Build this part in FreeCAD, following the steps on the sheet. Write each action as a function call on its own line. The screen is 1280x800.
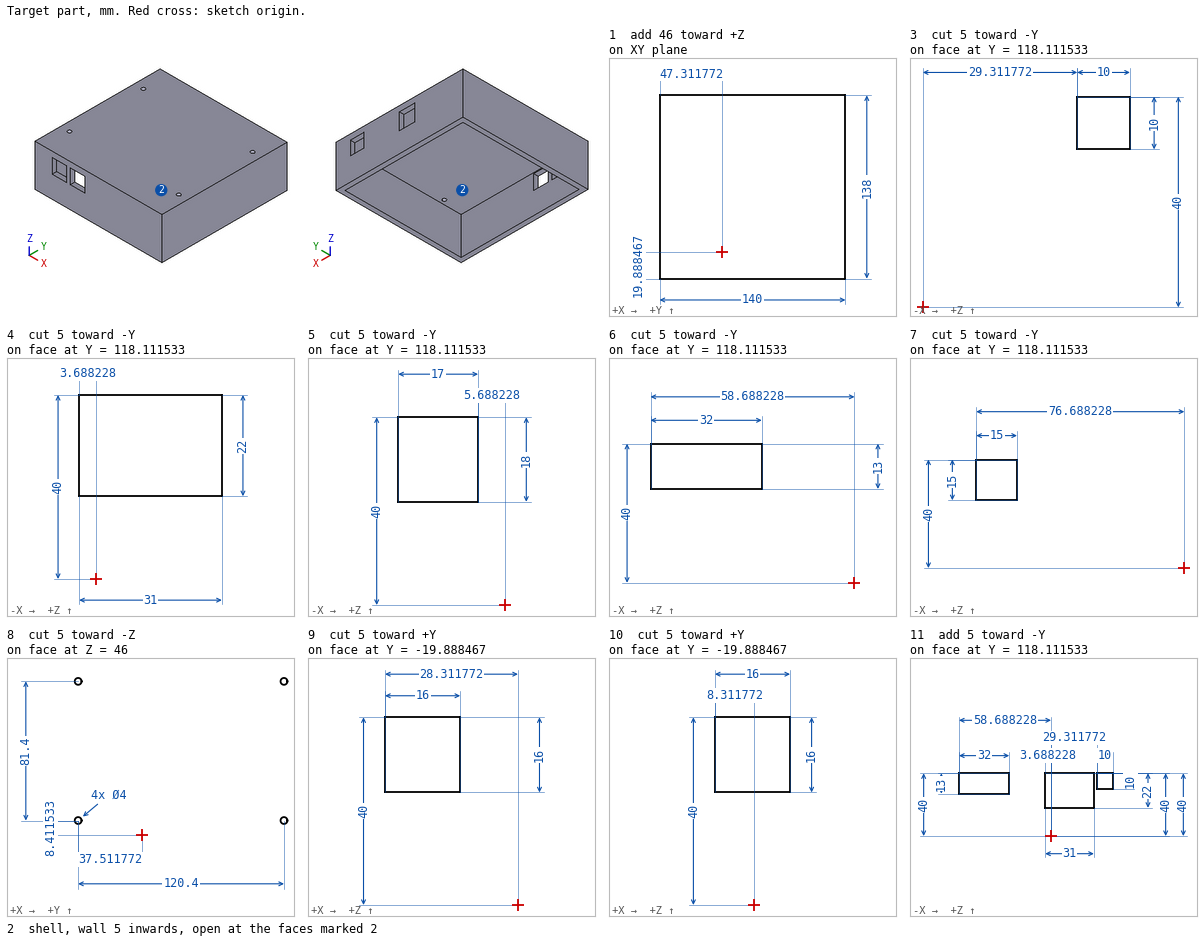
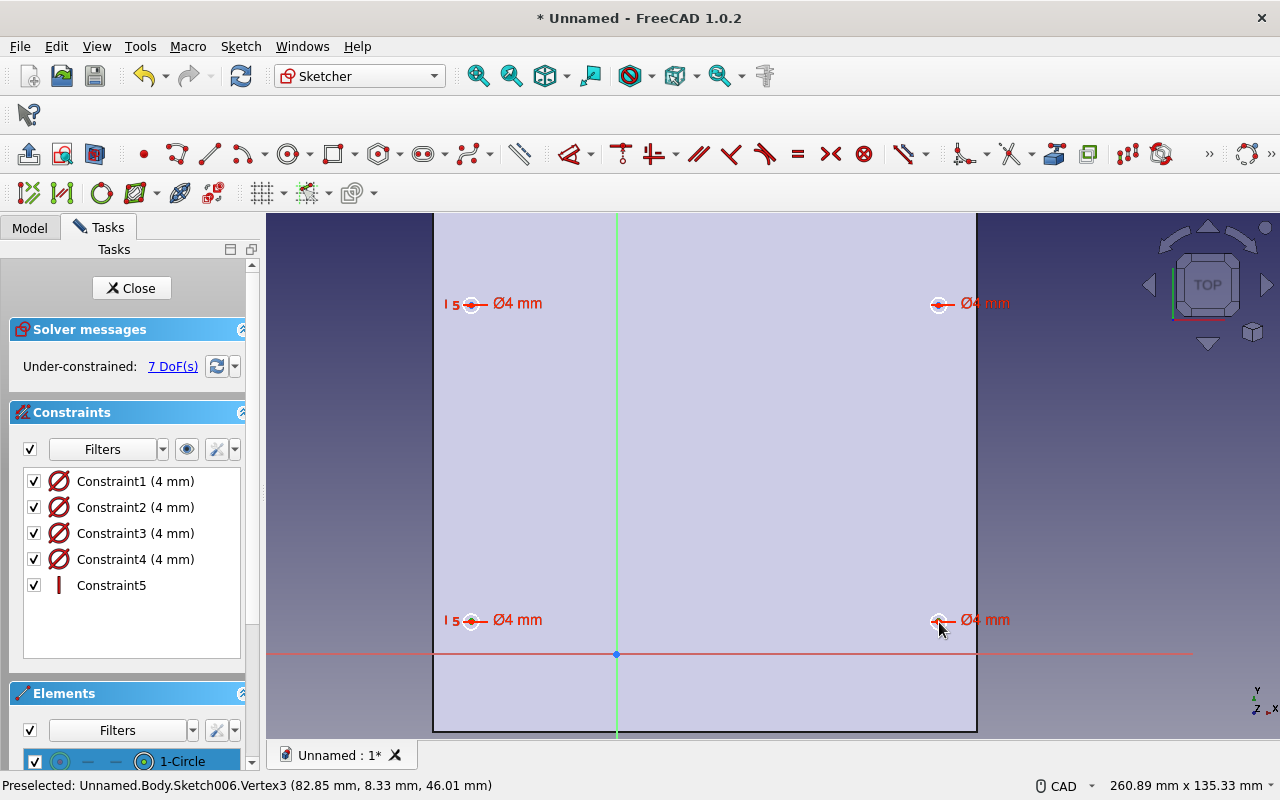
key(h)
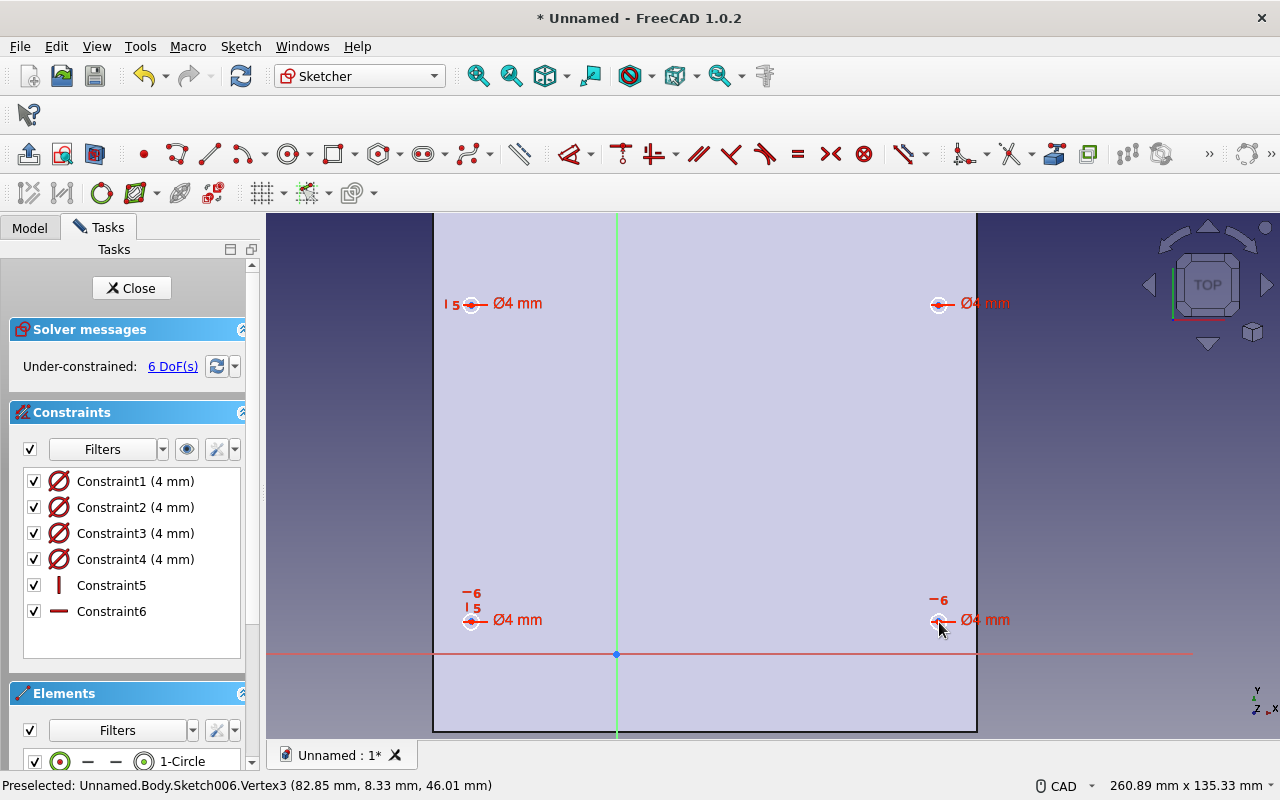
click(939, 622)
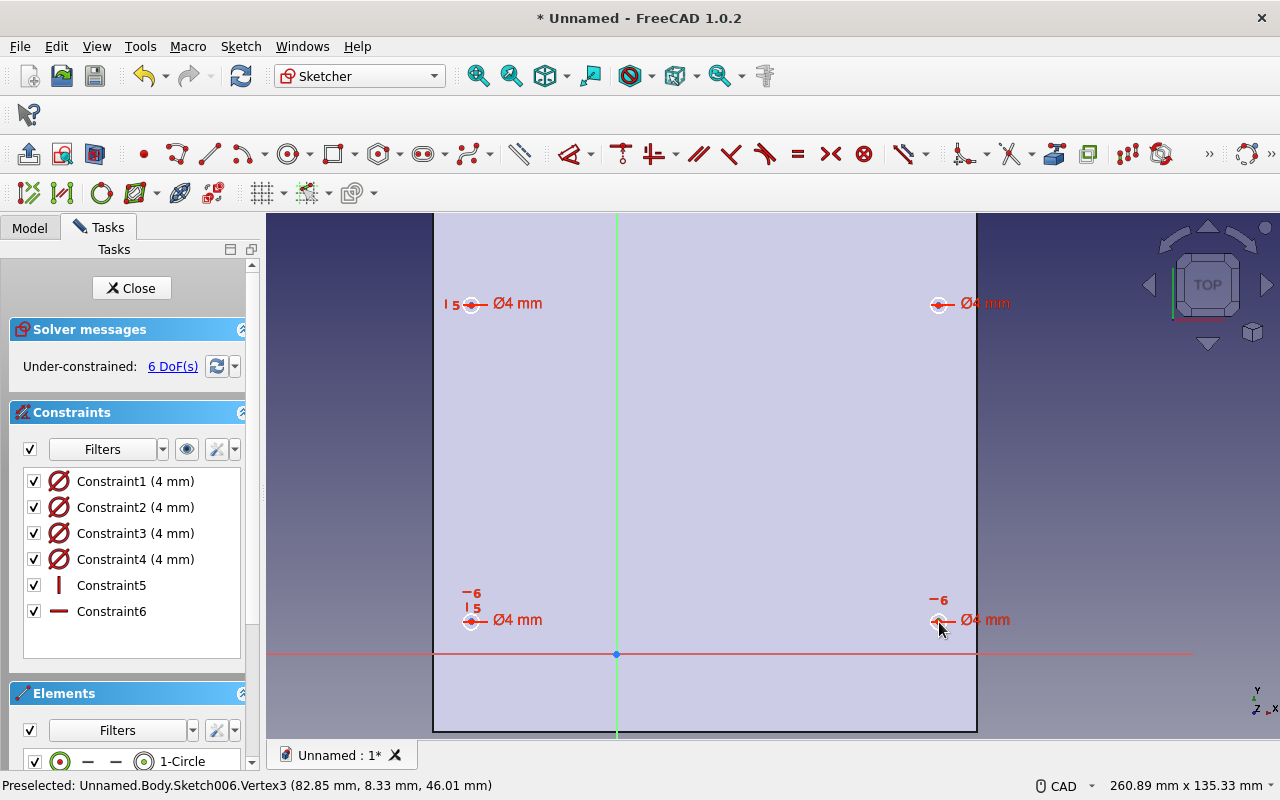
click(939, 305)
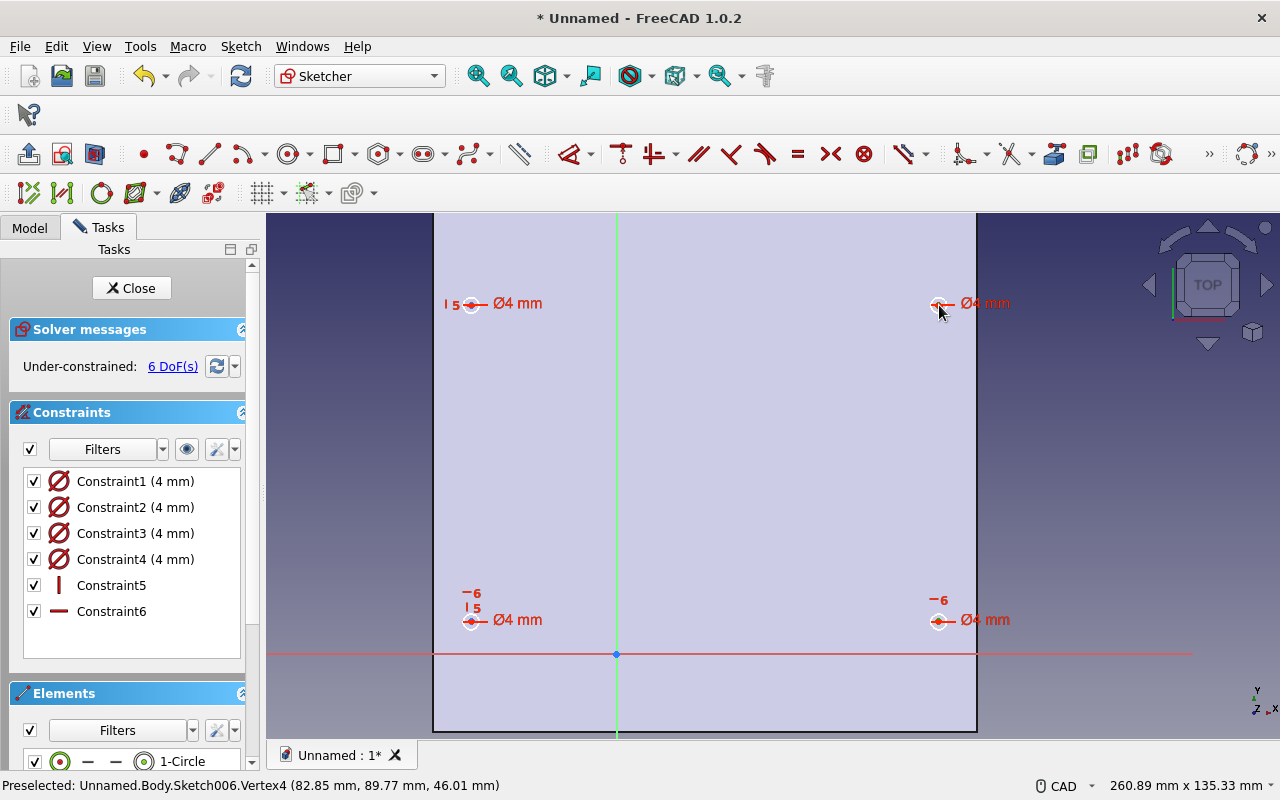
key(v)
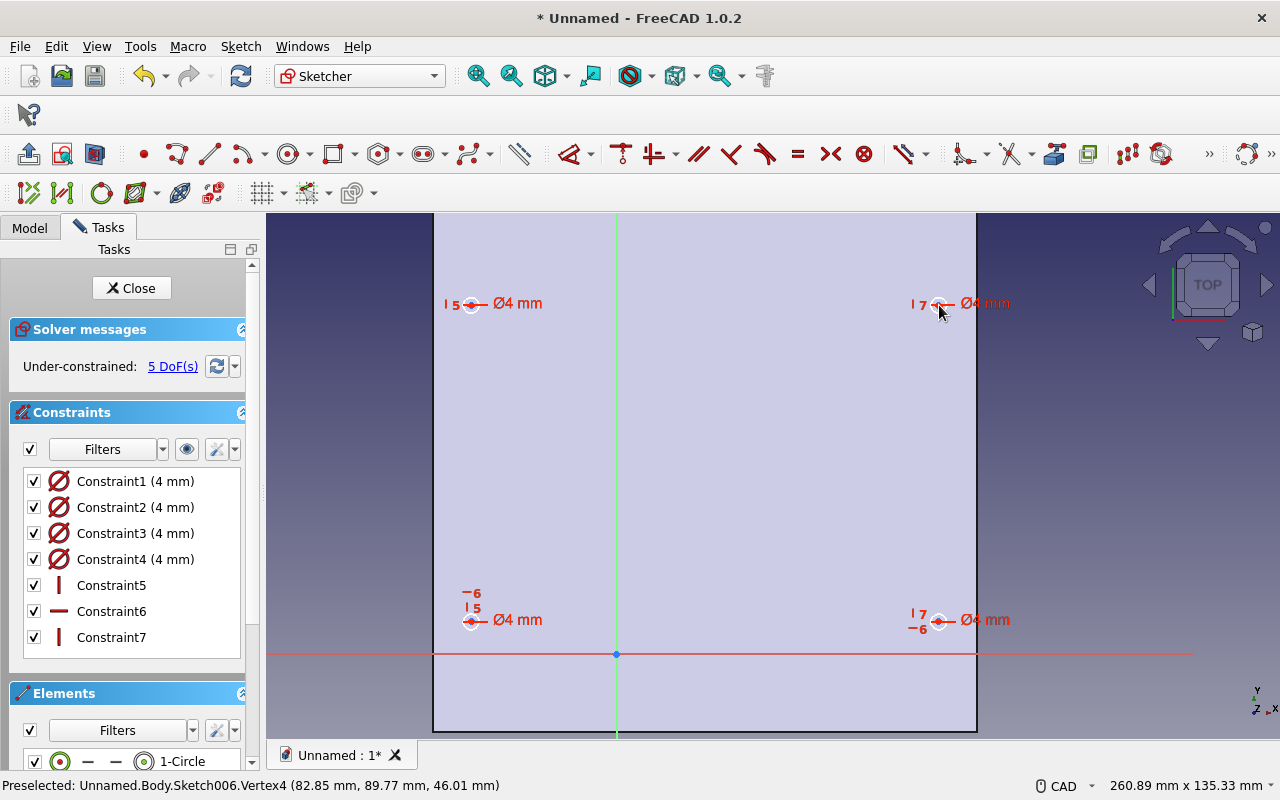
click(471, 305)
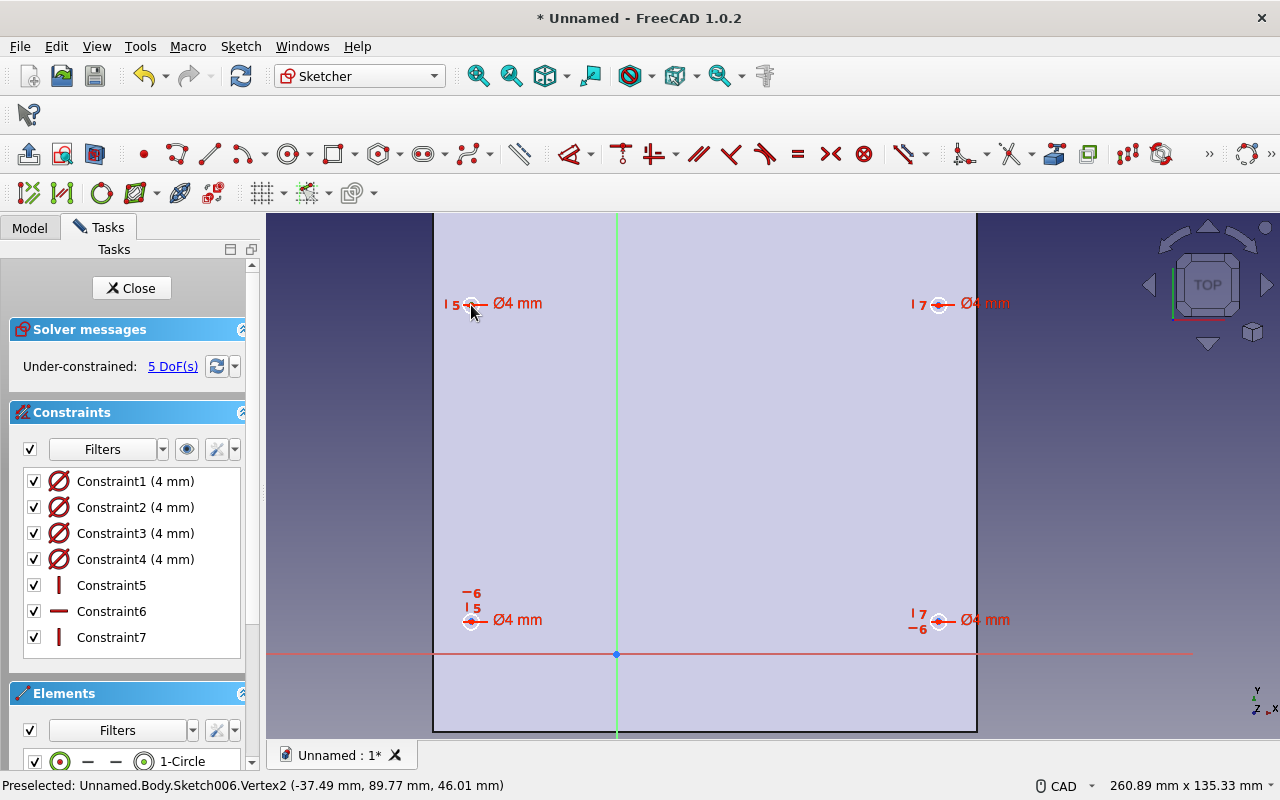
click(939, 305)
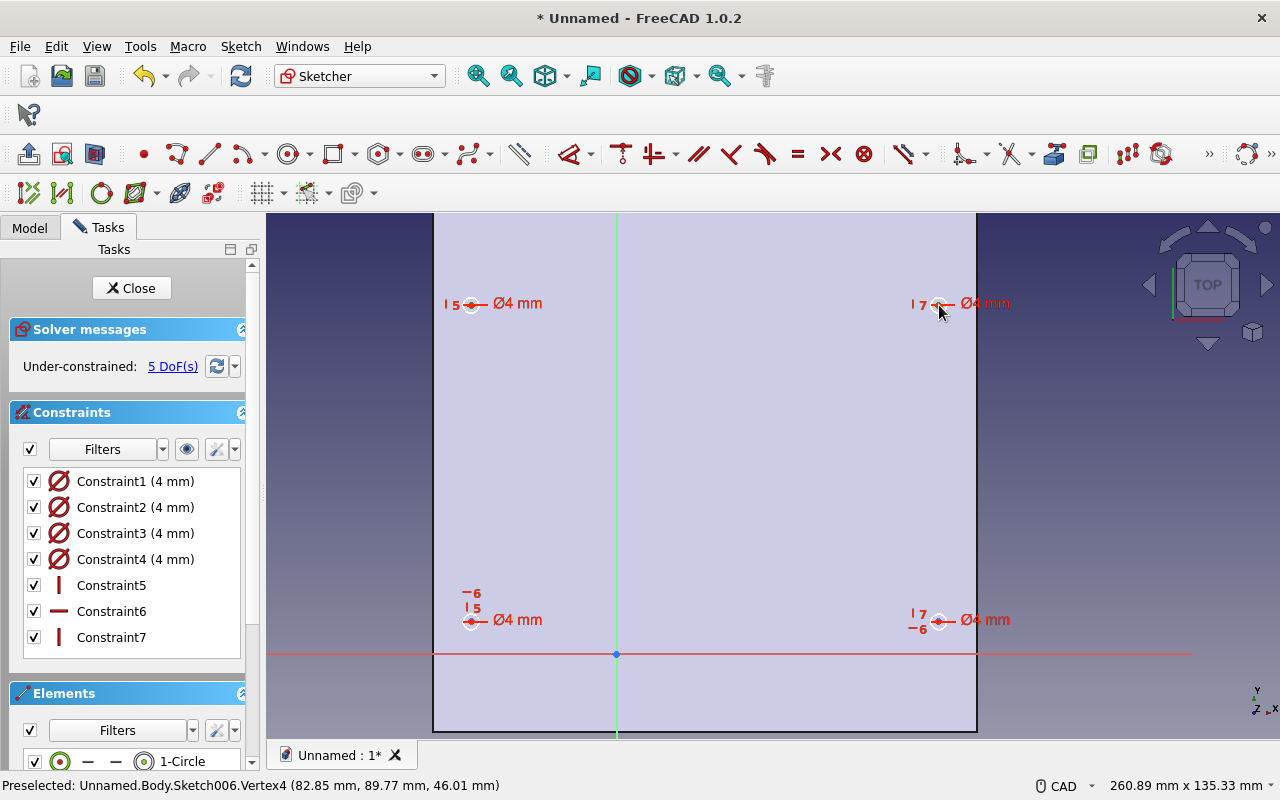
key(h)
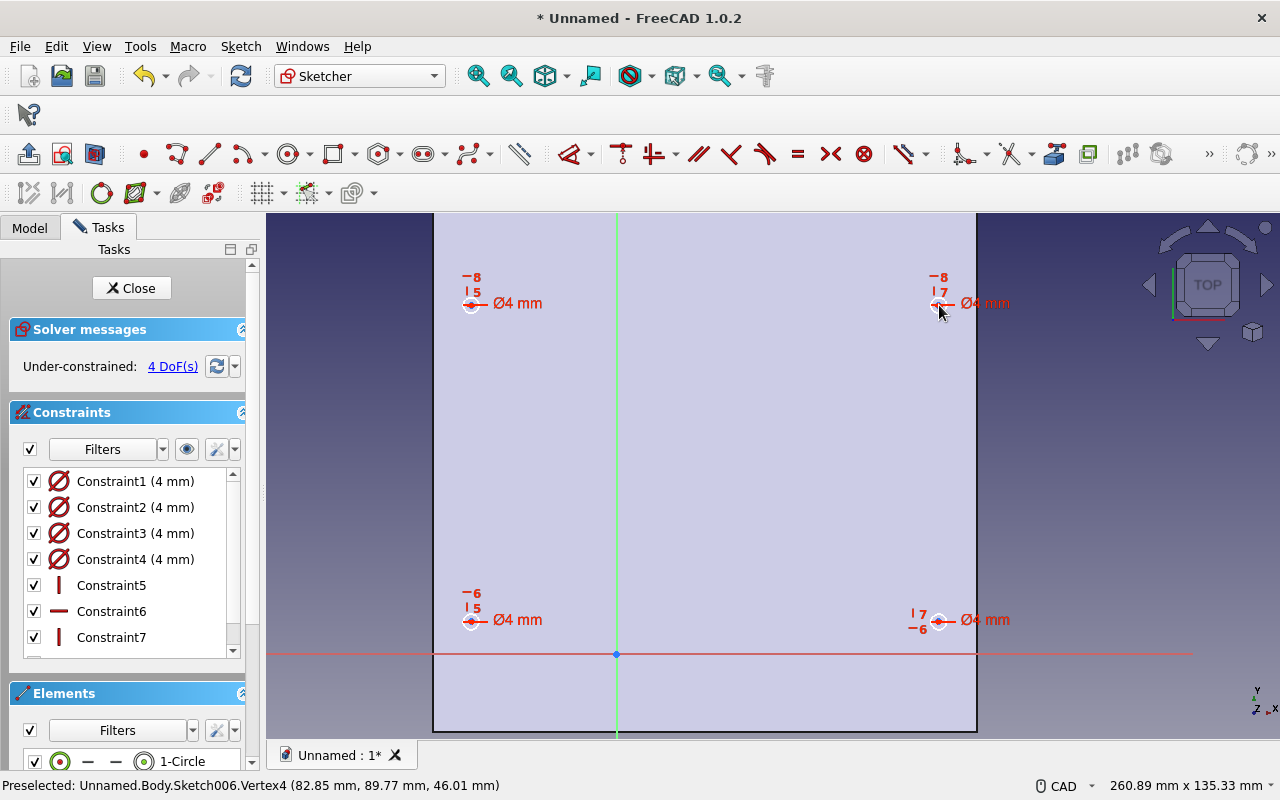
click(568, 154)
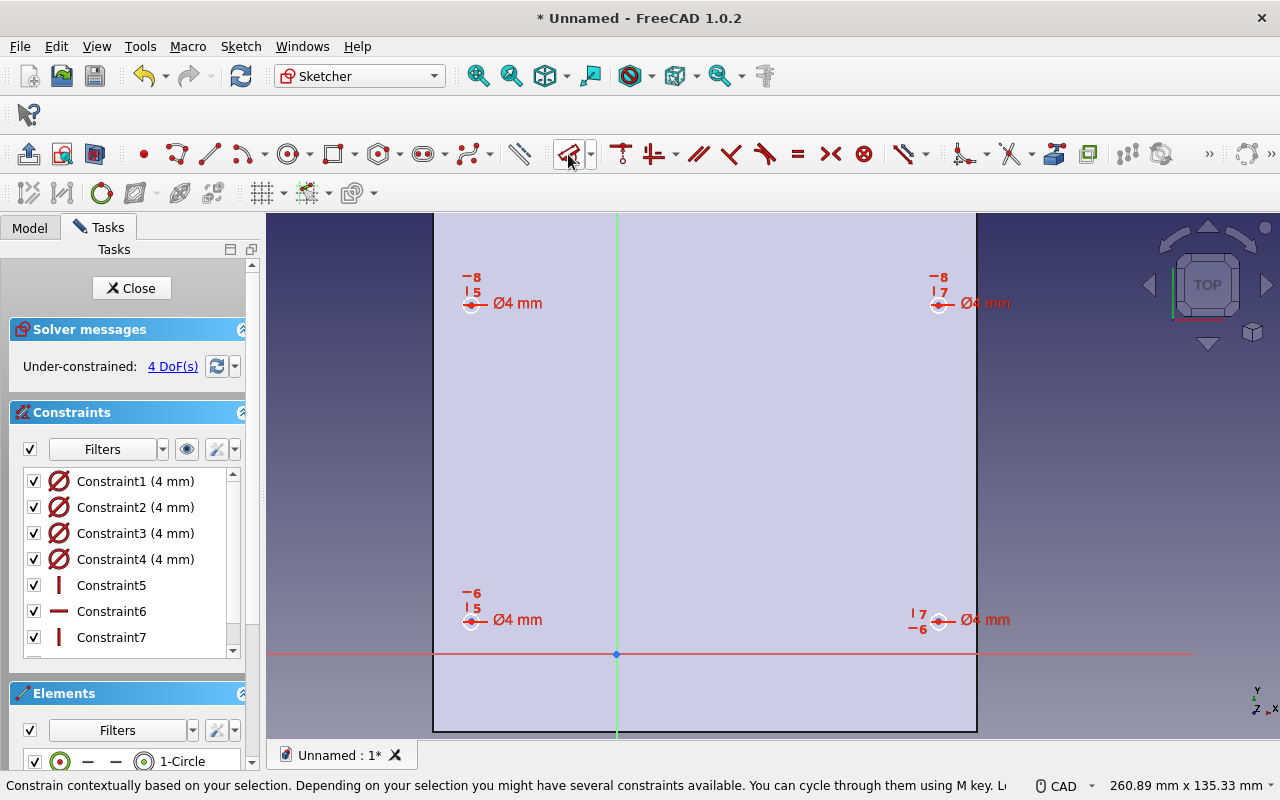
click(471, 622)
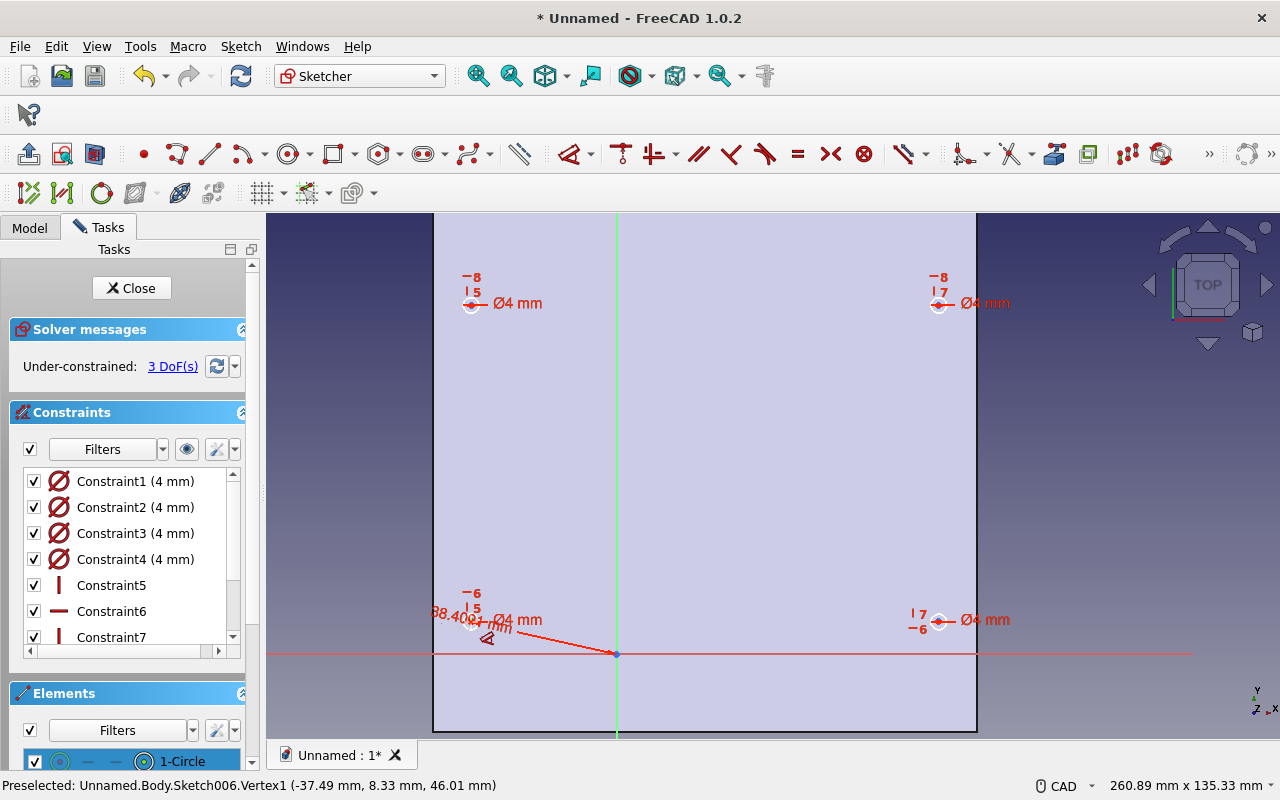
click(471, 305)
click(437, 464)